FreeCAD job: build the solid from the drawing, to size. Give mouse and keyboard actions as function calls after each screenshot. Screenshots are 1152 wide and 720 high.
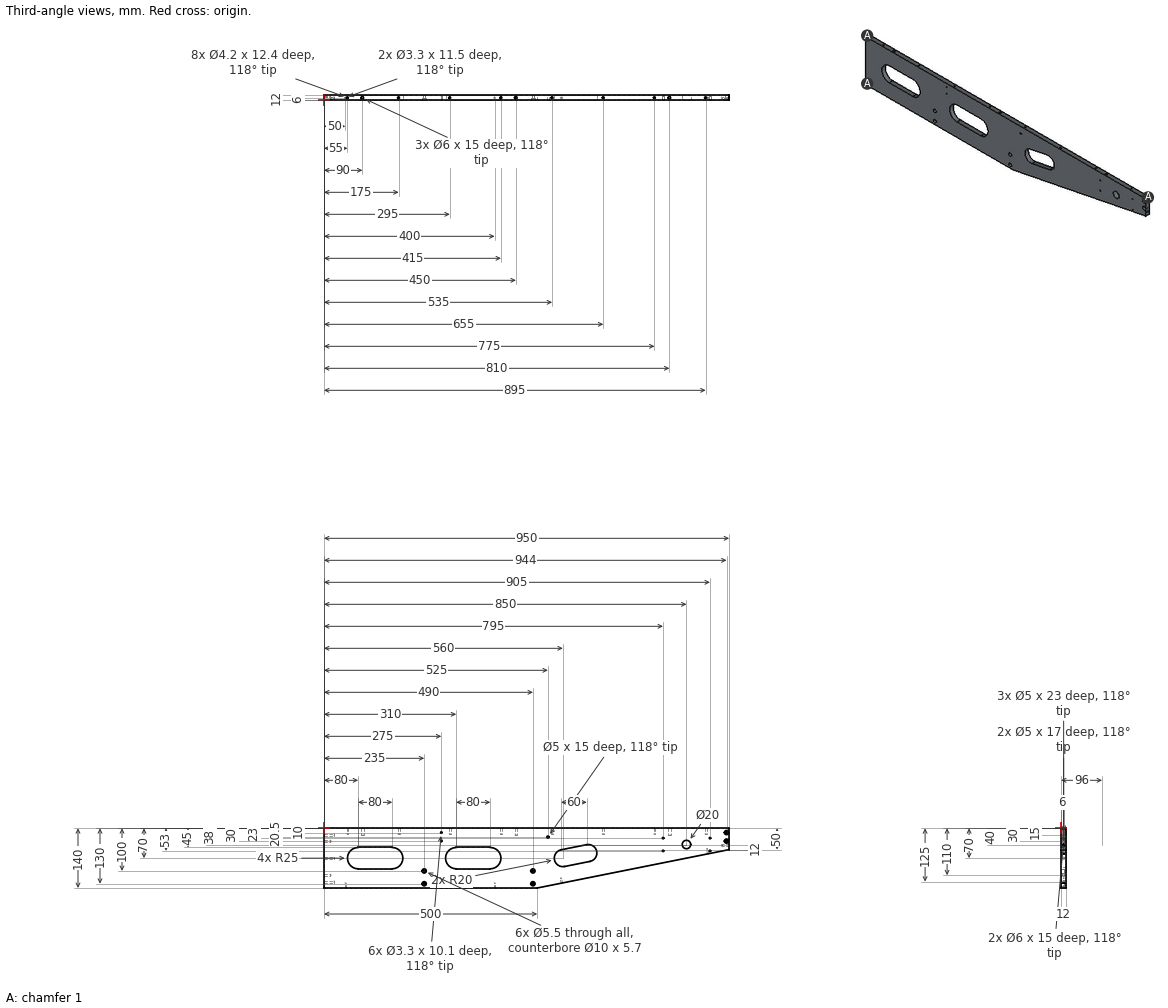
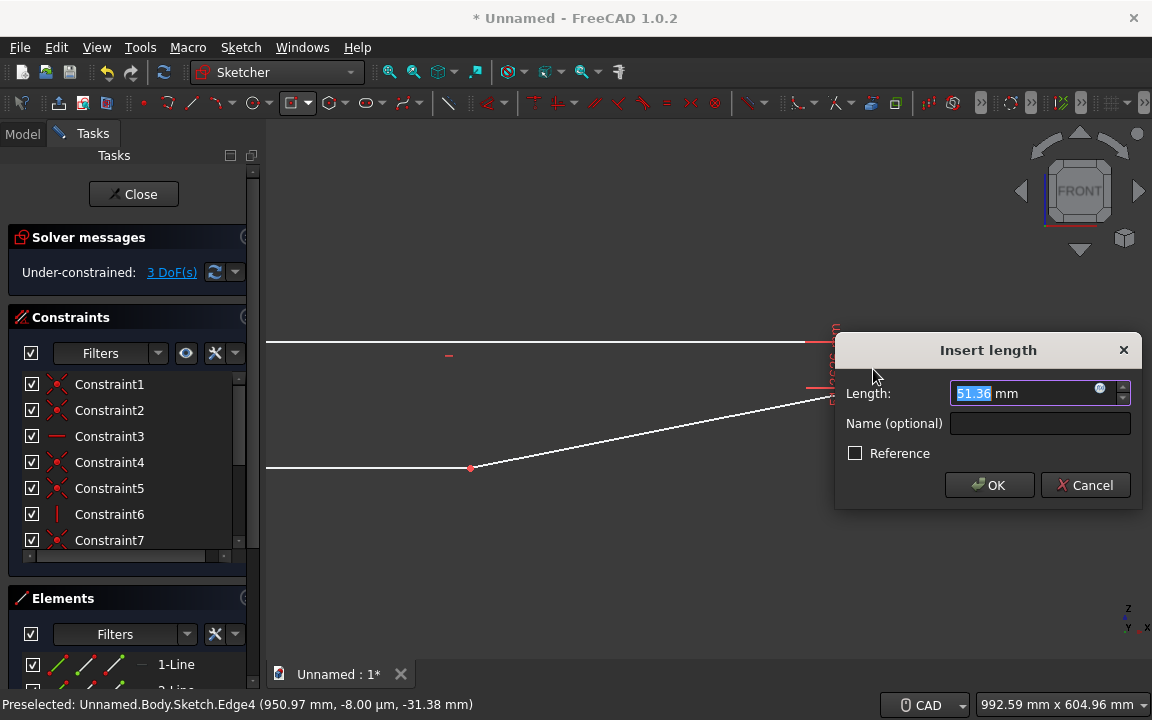
text(50)
key(Return)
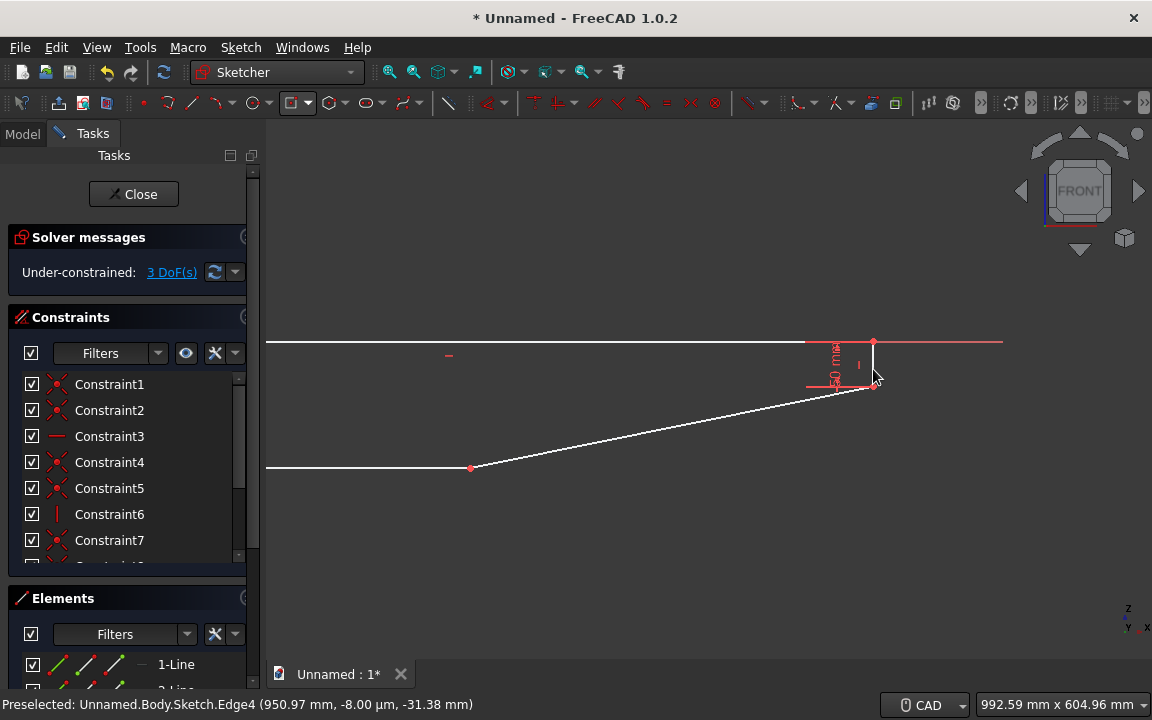
scroll(874, 370, down, 3)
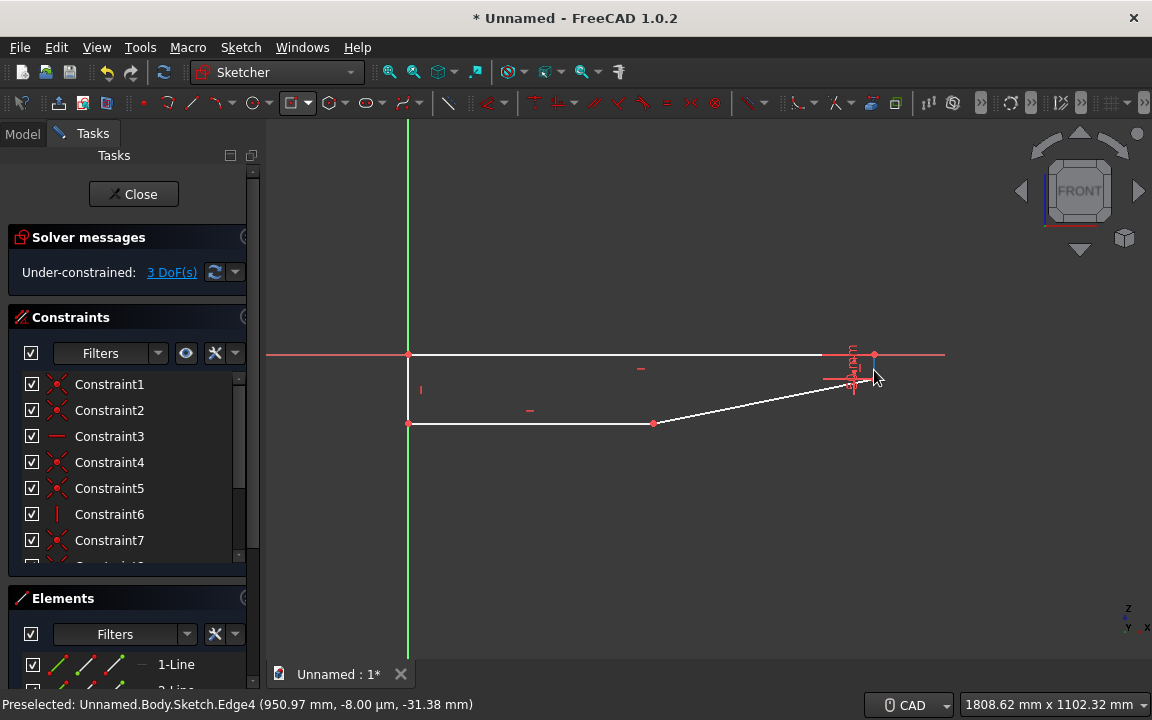
click(408, 376)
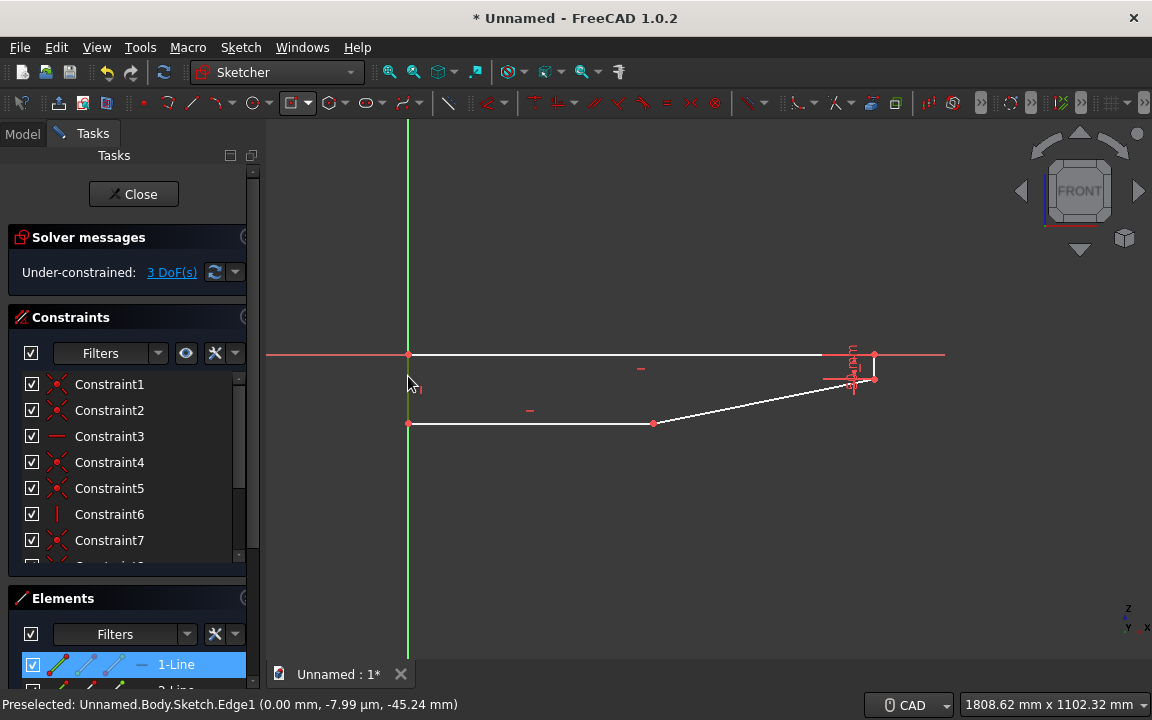
key(i)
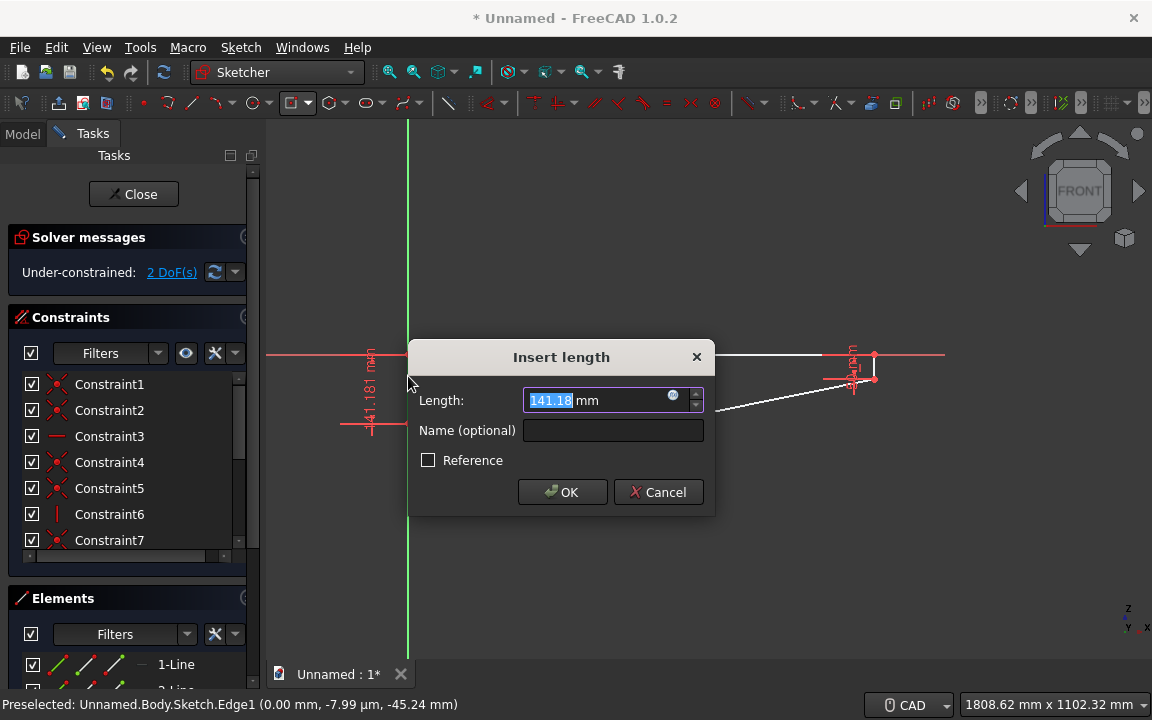
text(140)
key(Return)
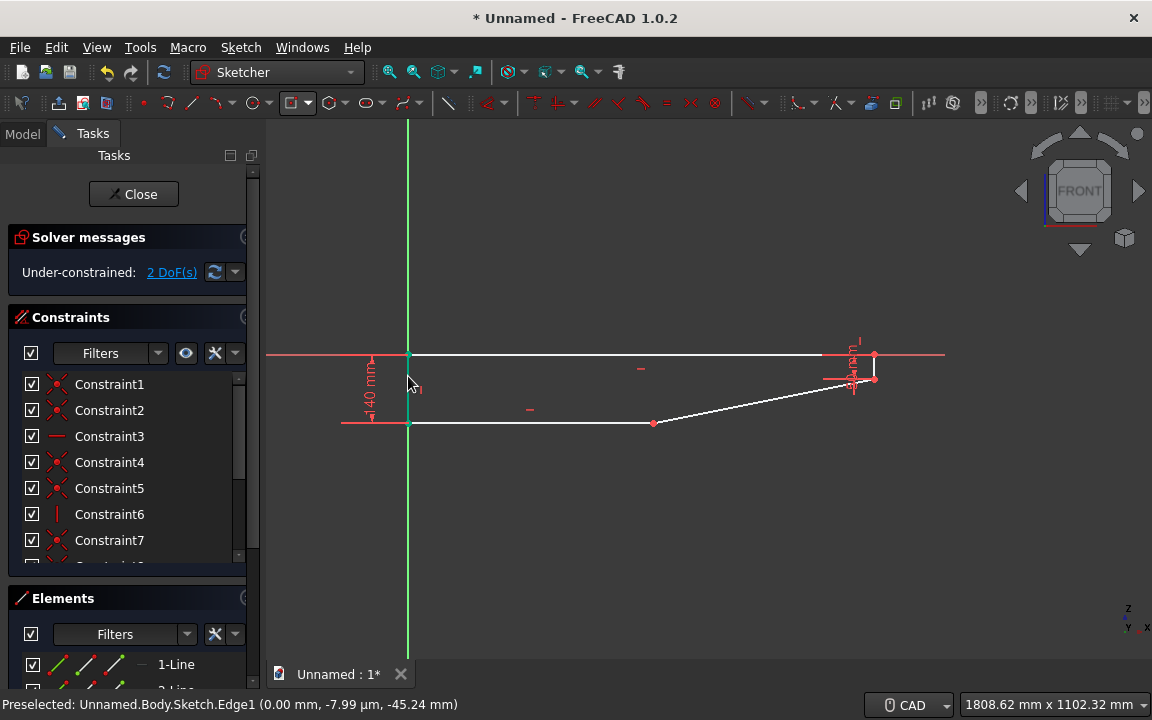
click(482, 423)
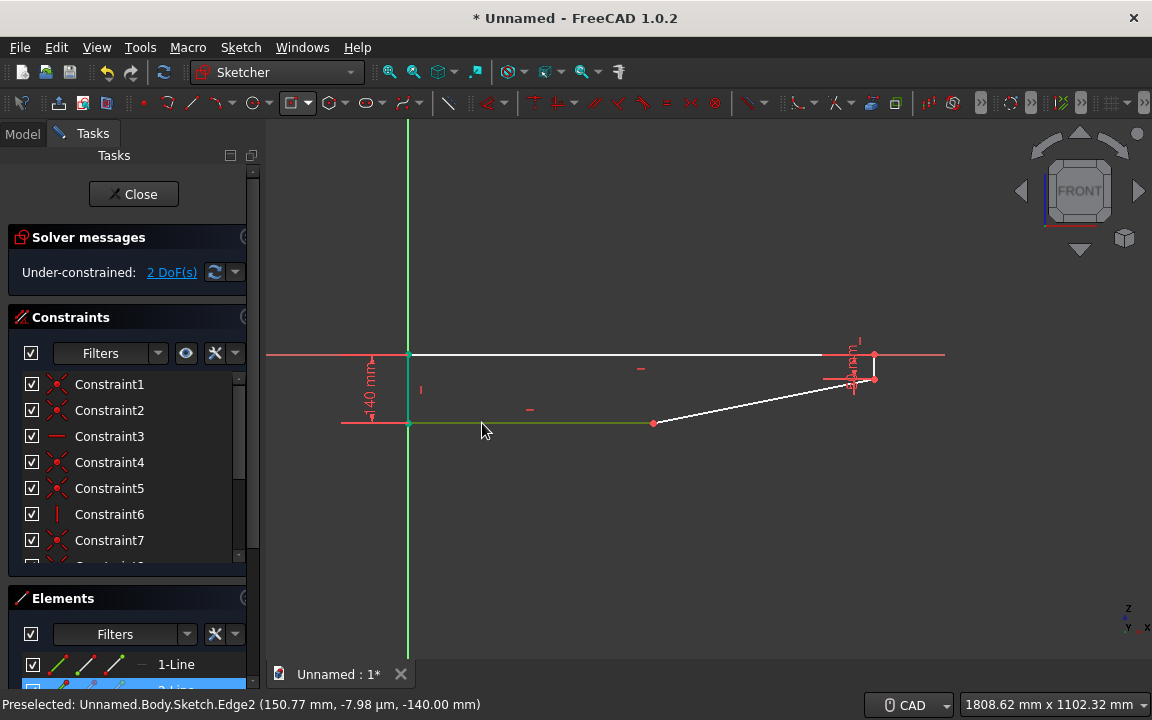
click(506, 104)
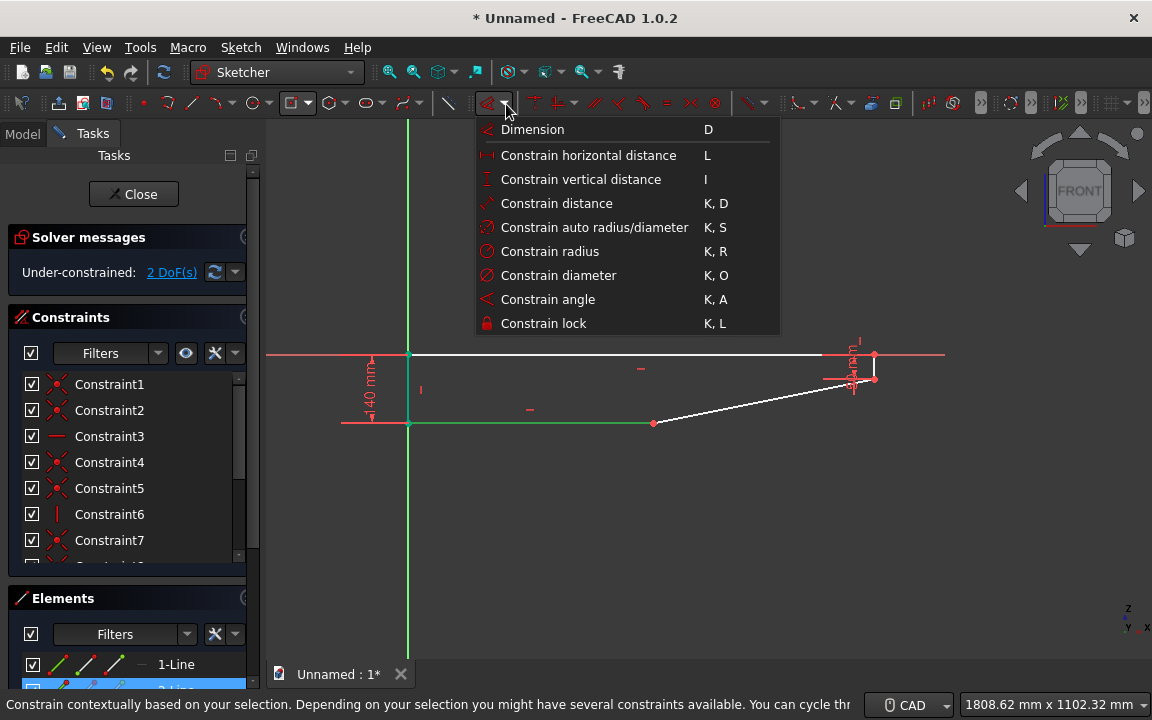
click(628, 155)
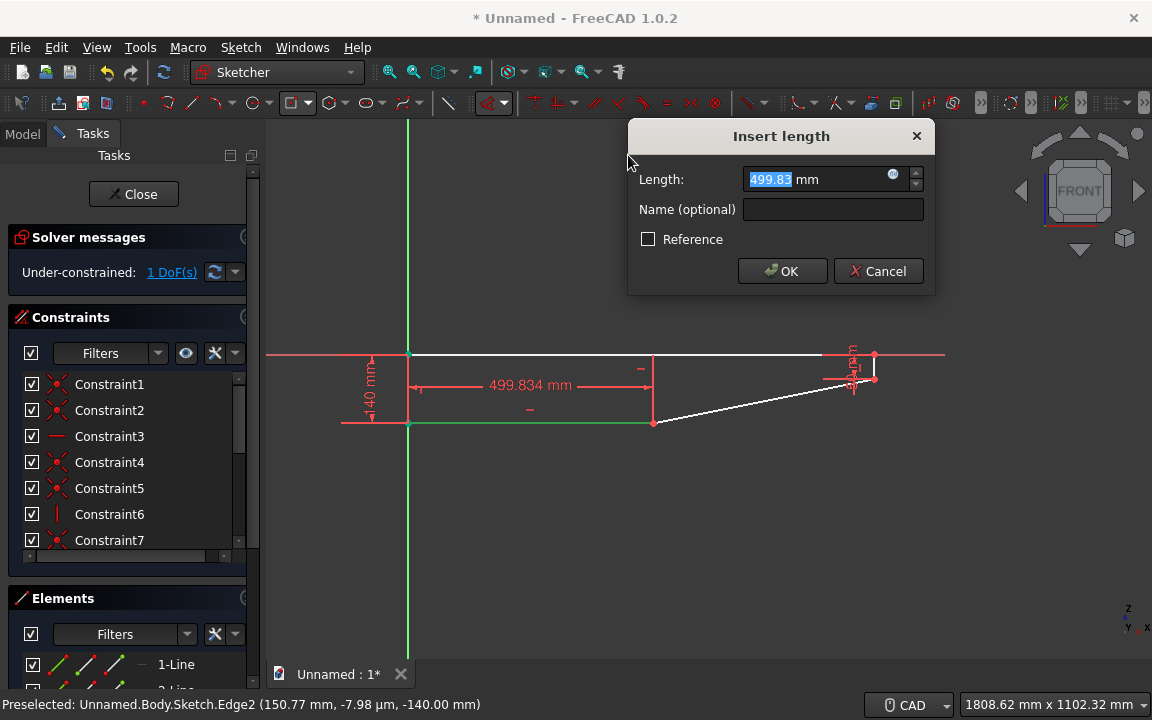
text(500)
key(Return)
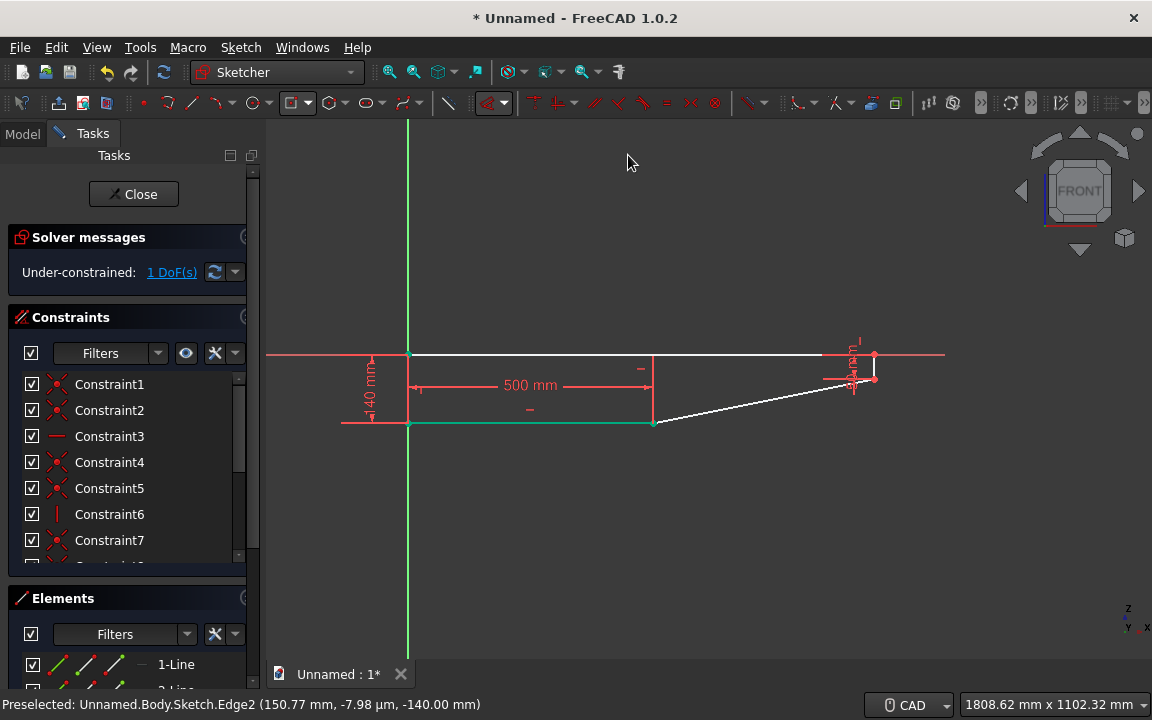
click(734, 355)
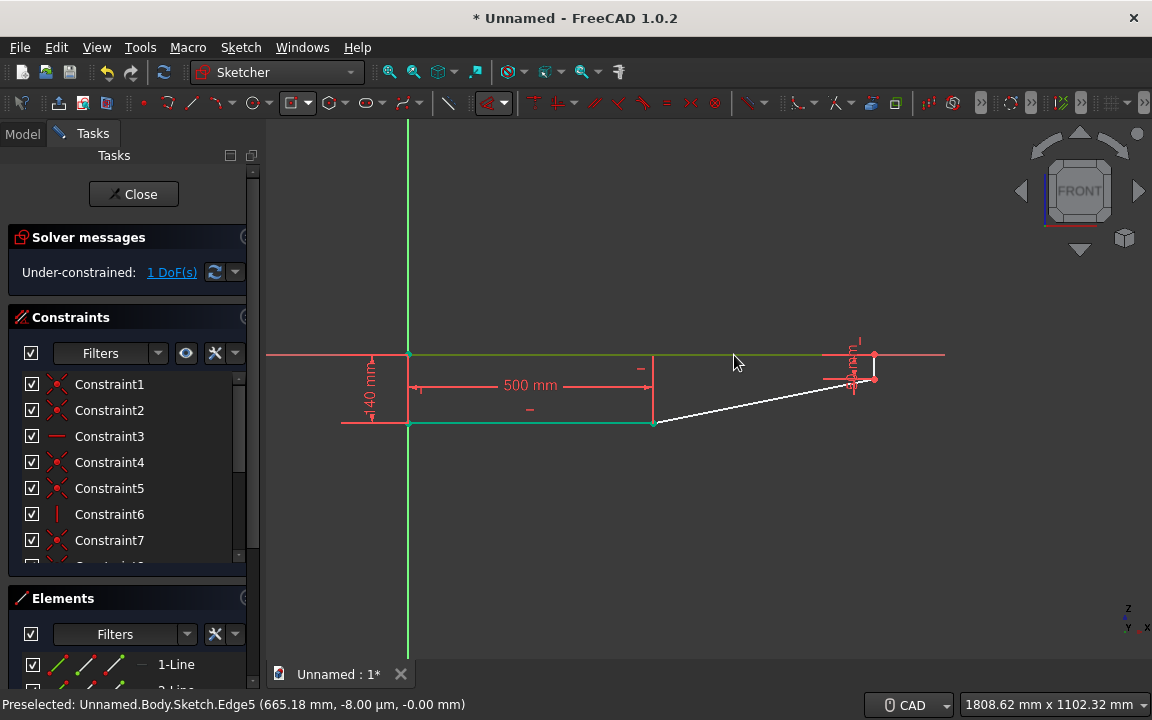
key(l)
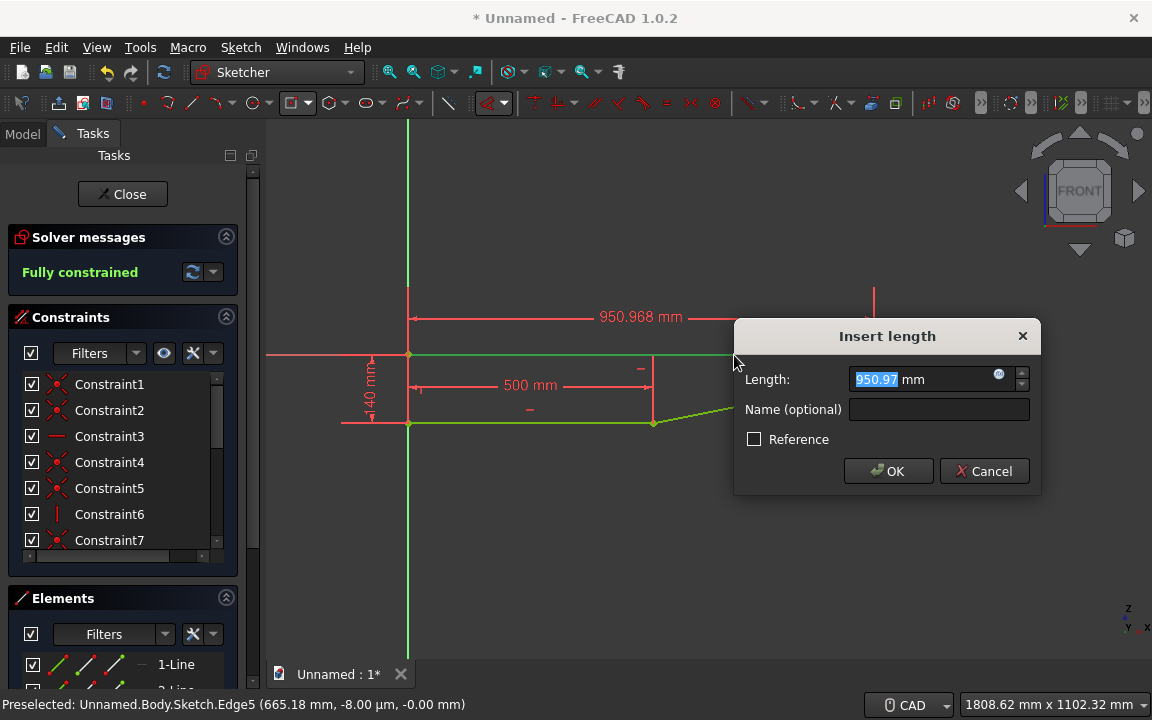
text(950)
key(Return)